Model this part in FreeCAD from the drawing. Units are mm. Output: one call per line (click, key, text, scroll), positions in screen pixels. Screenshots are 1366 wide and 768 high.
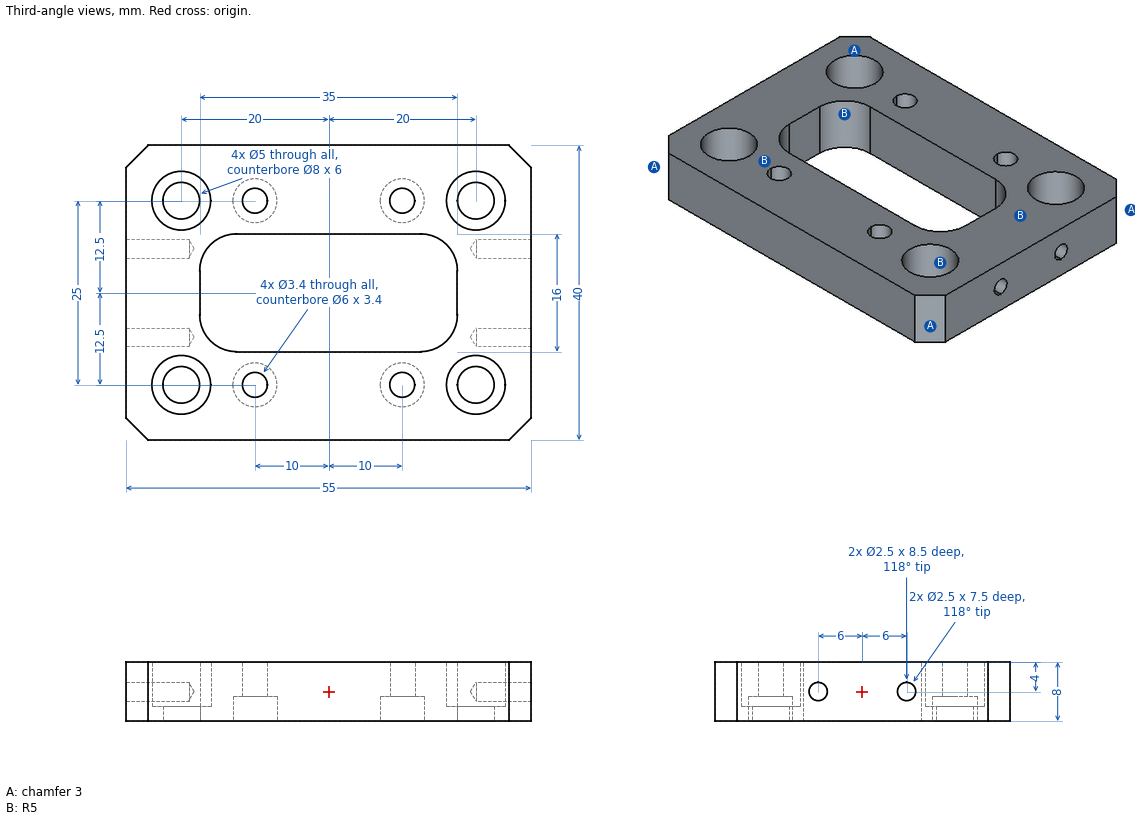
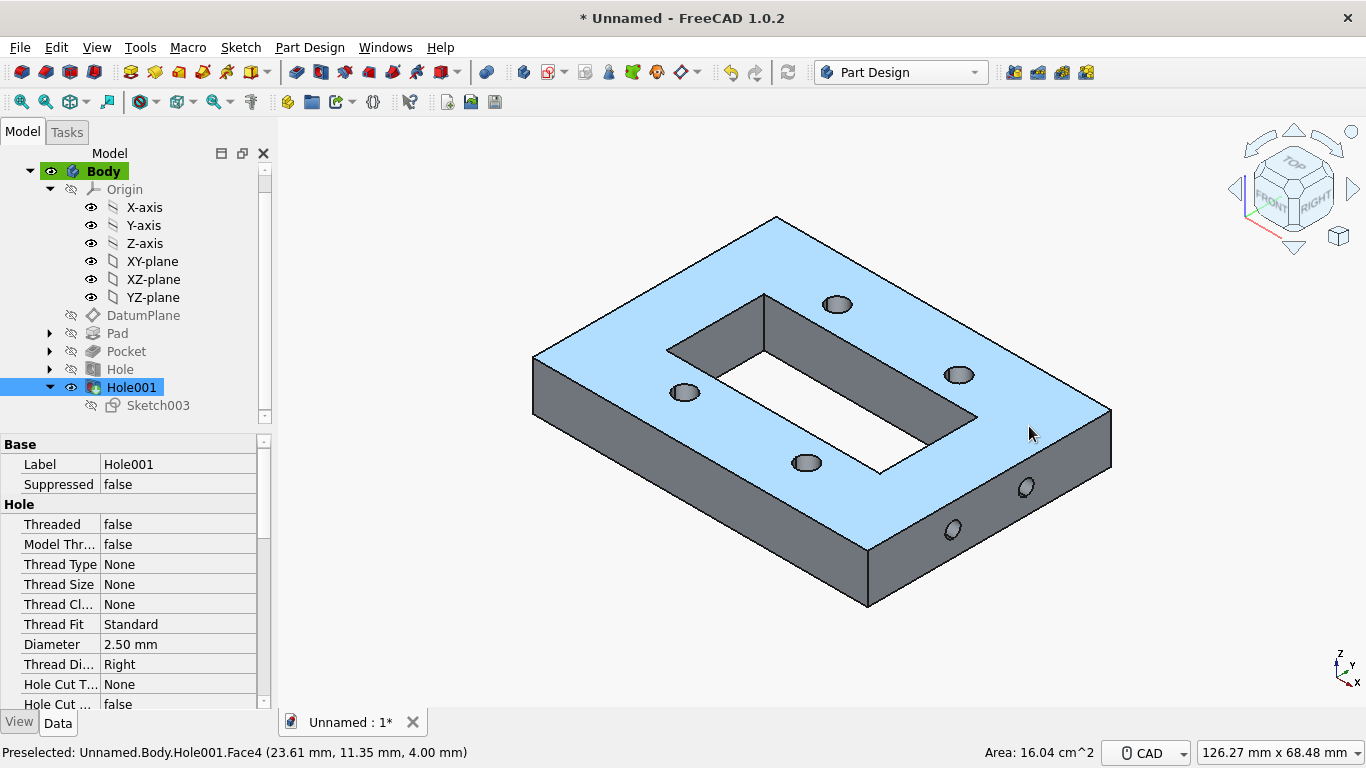
click(548, 72)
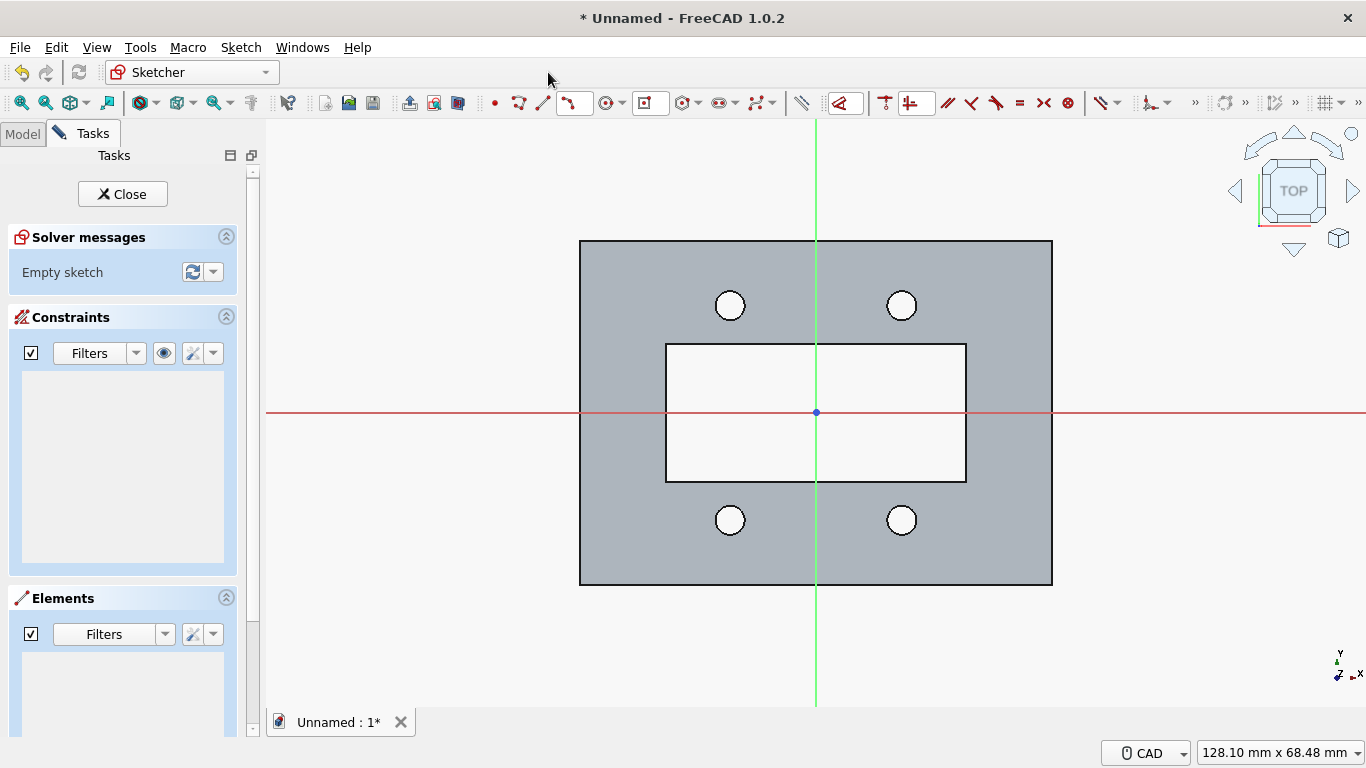
scroll(955, 413, up, 2)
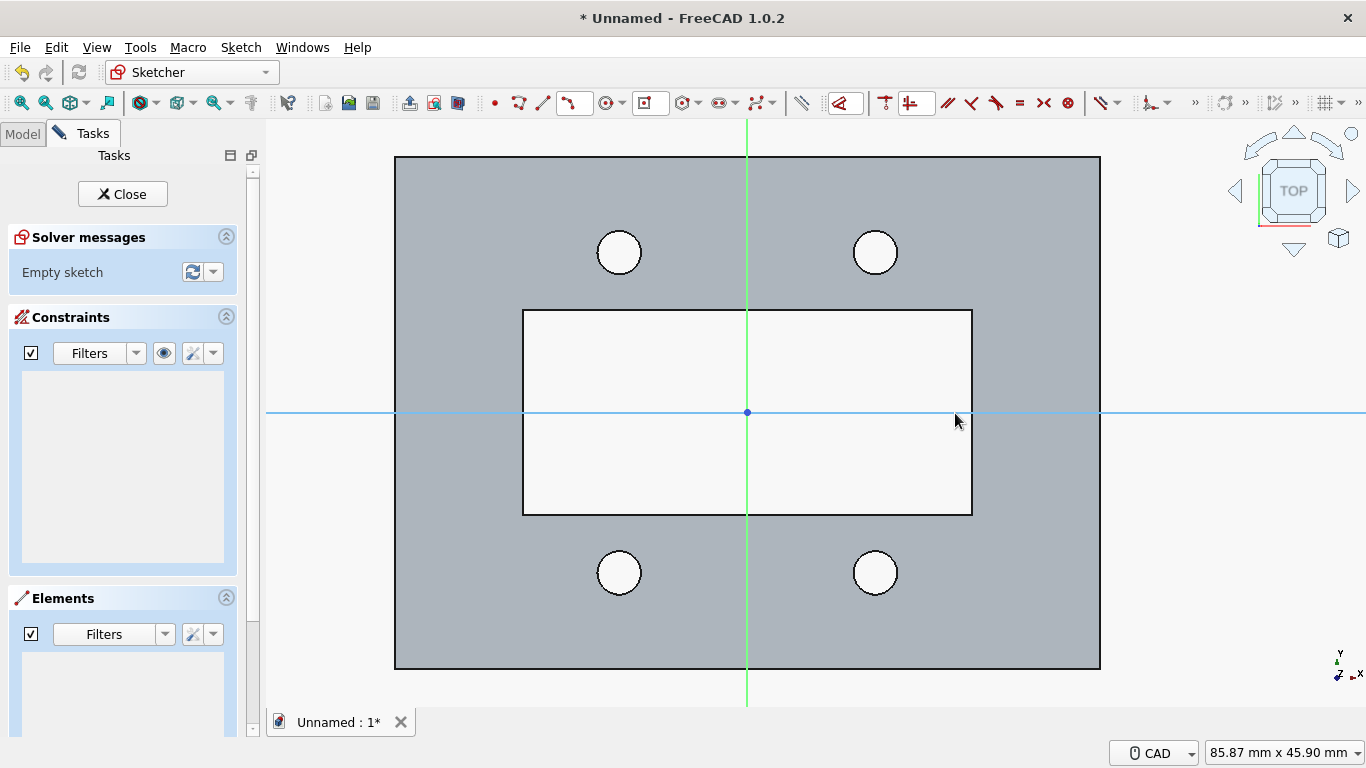
click(606, 104)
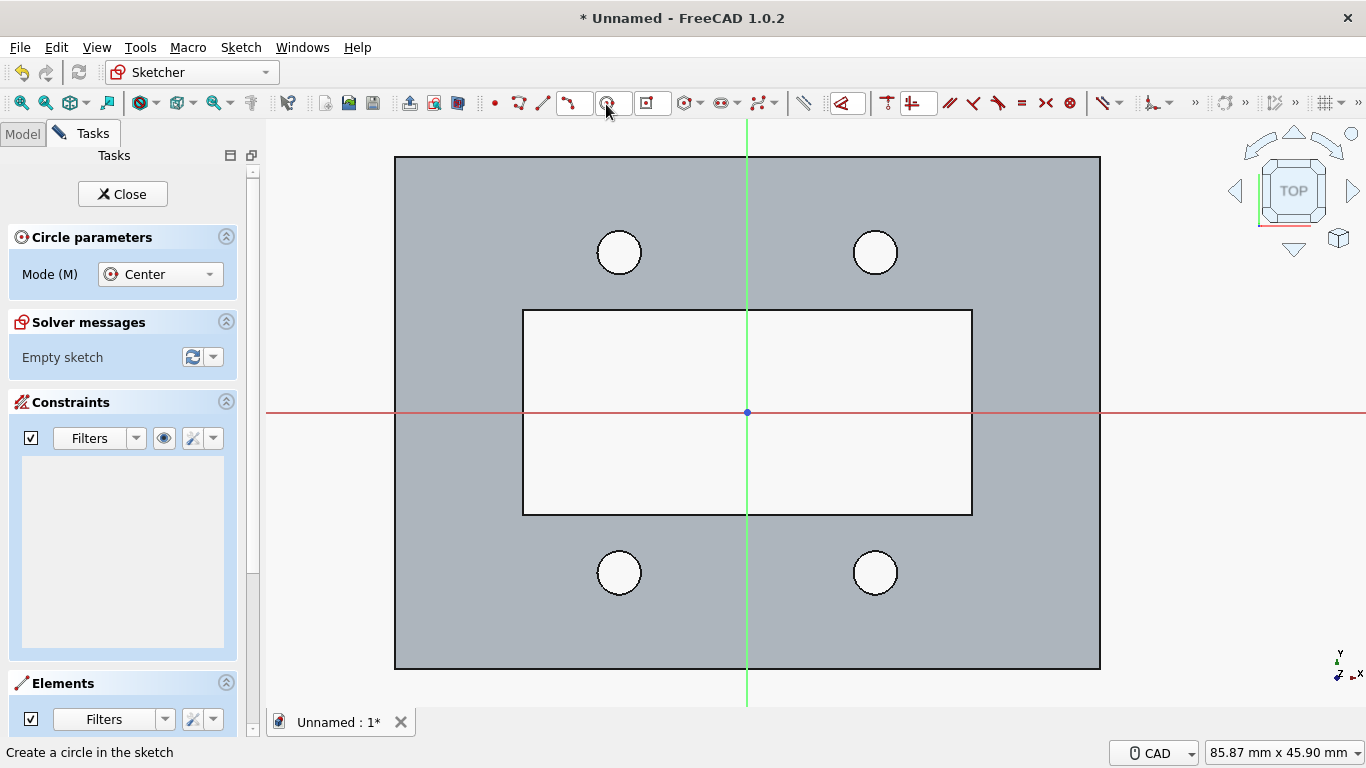
click(491, 253)
move(514, 230)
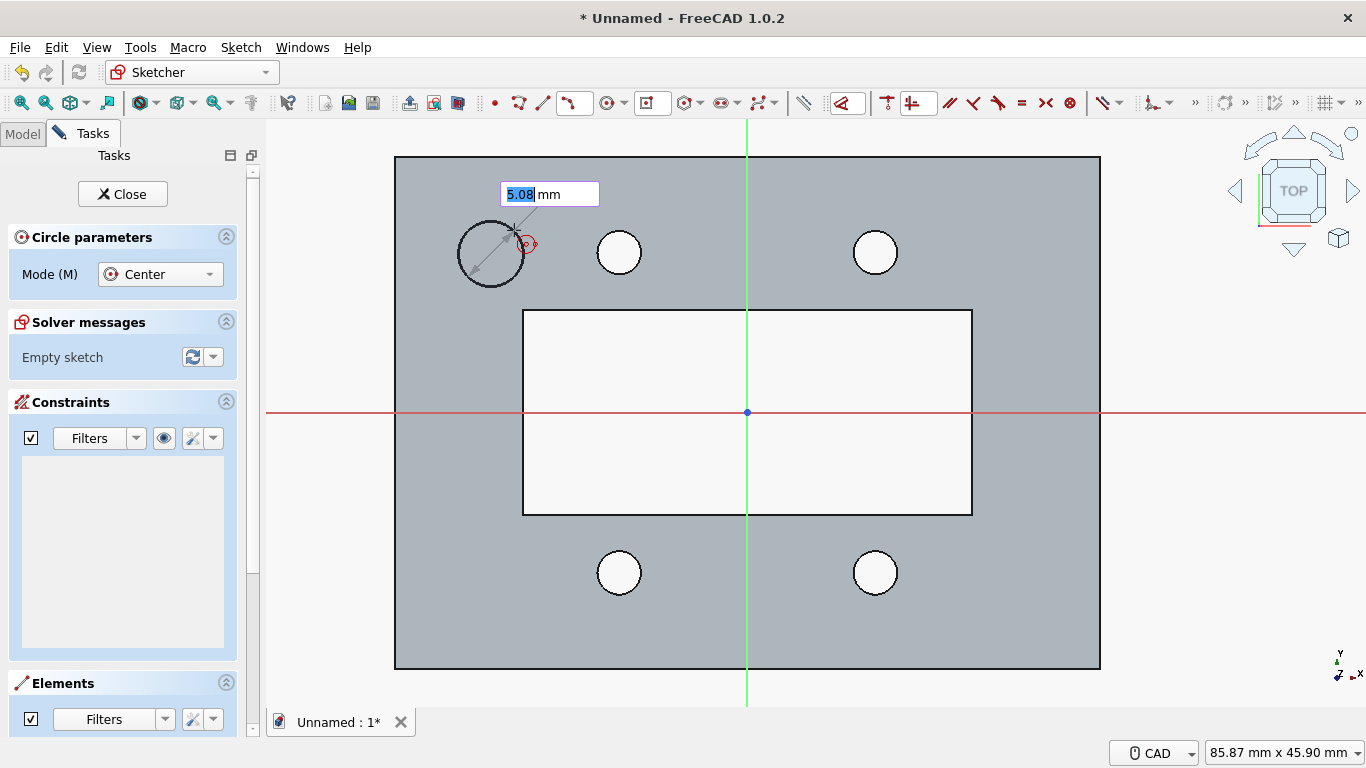
text(5)
key(Return)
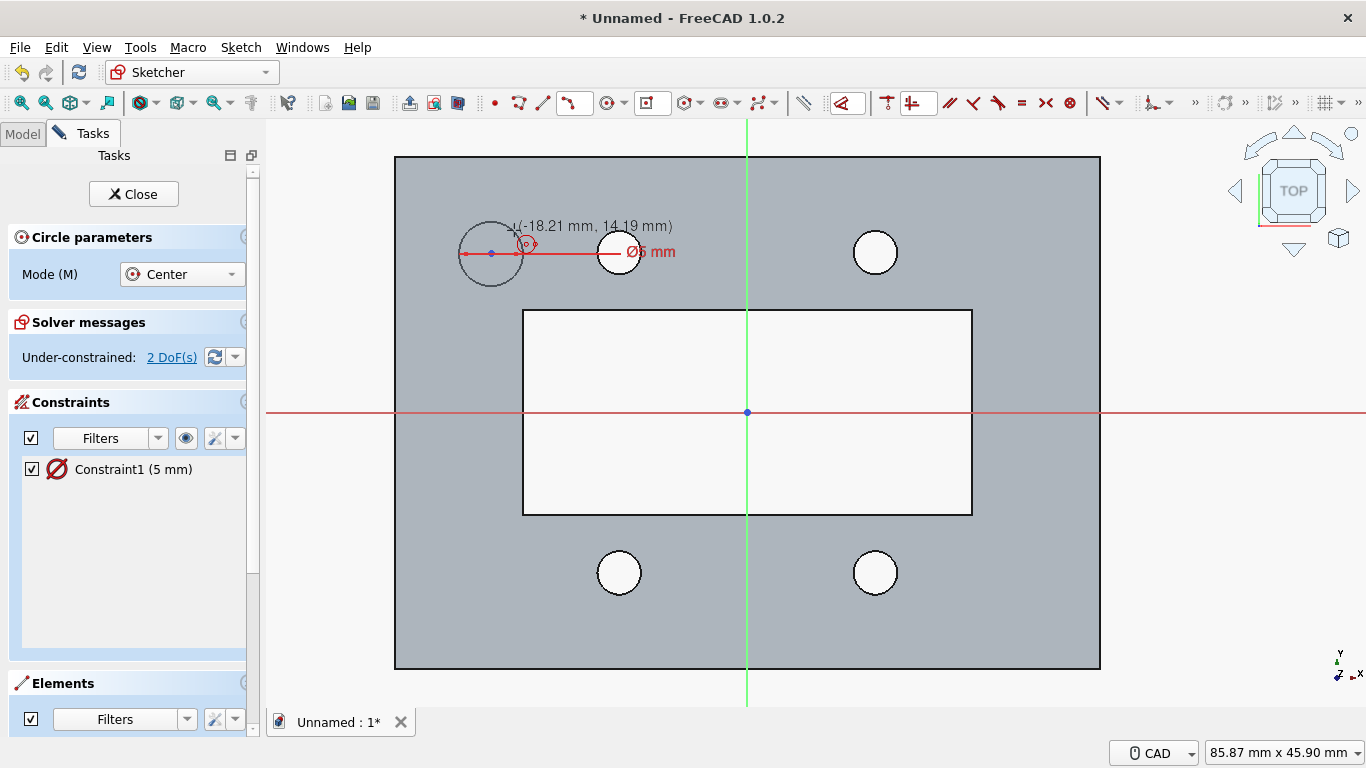
click(491, 573)
move(514, 550)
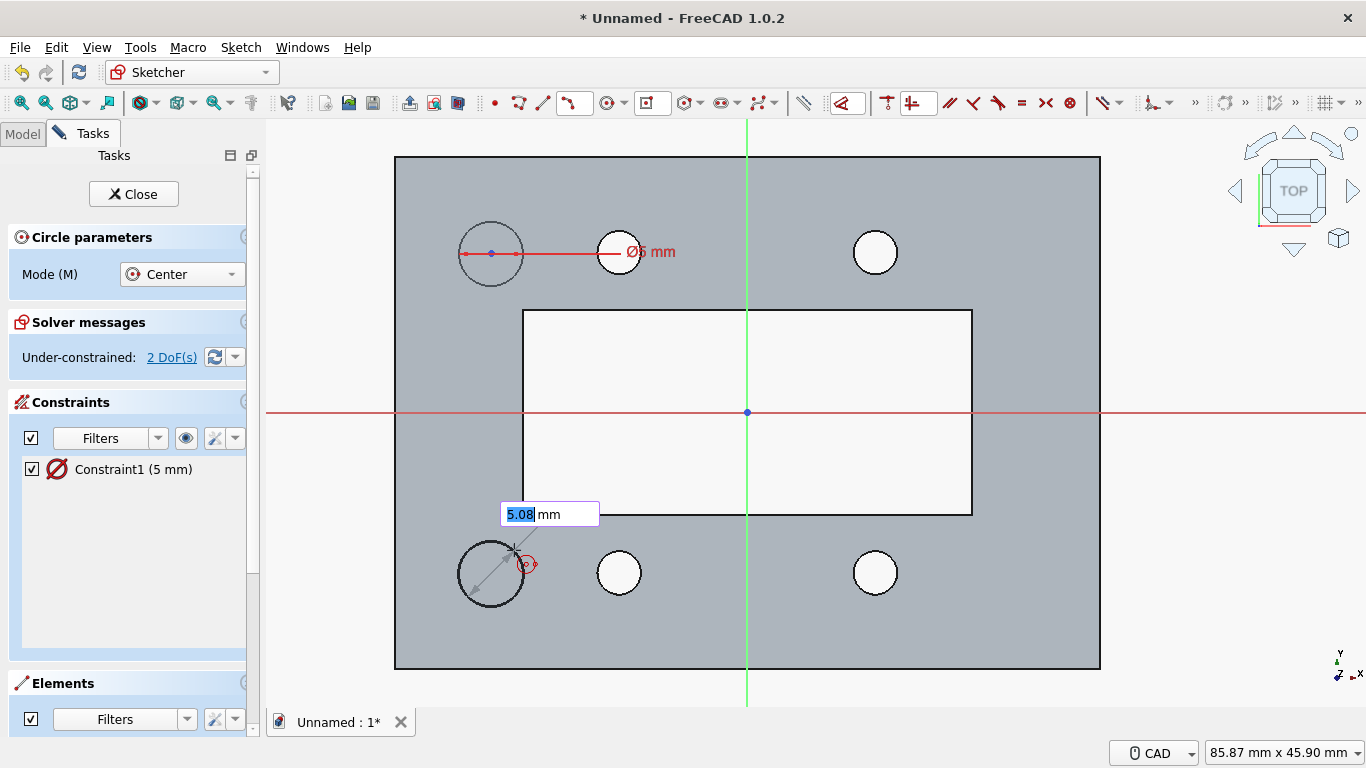
text(5)
key(Return)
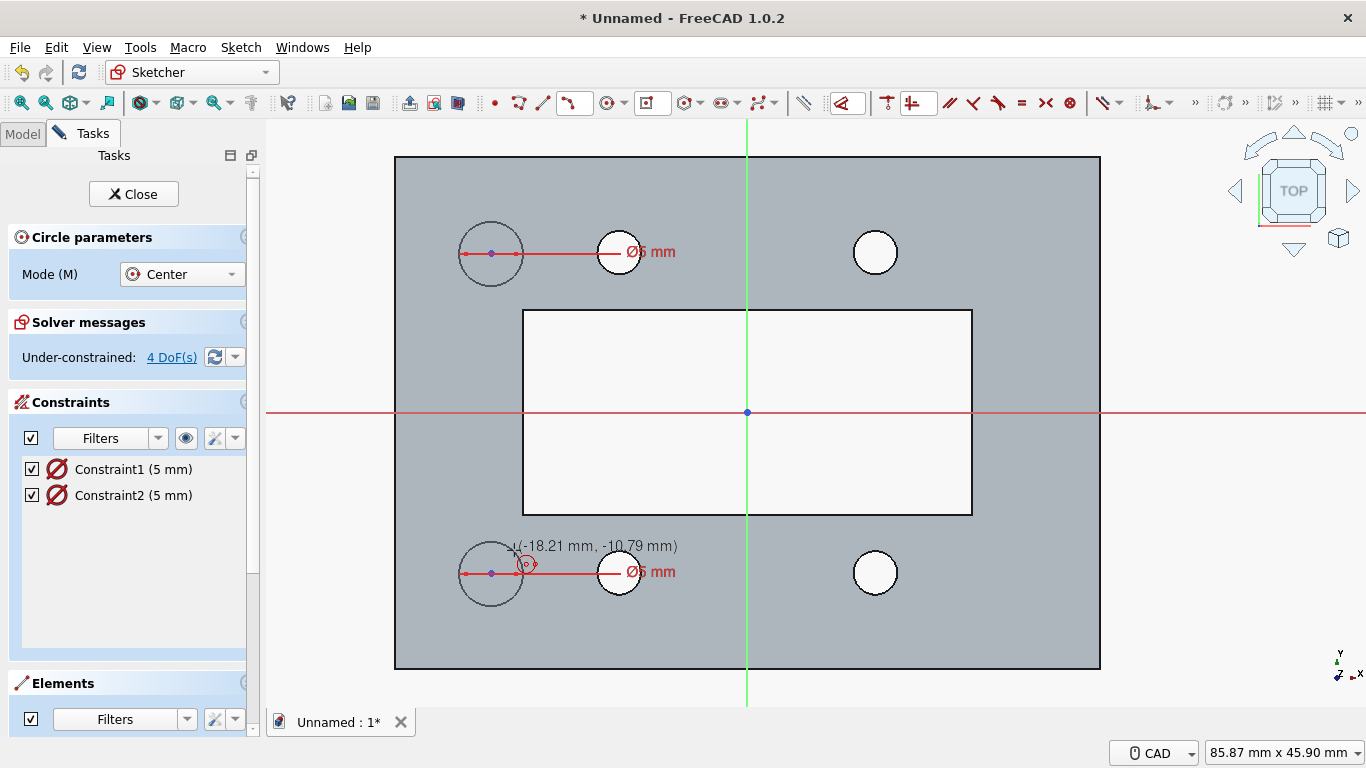
click(1004, 253)
move(1026, 230)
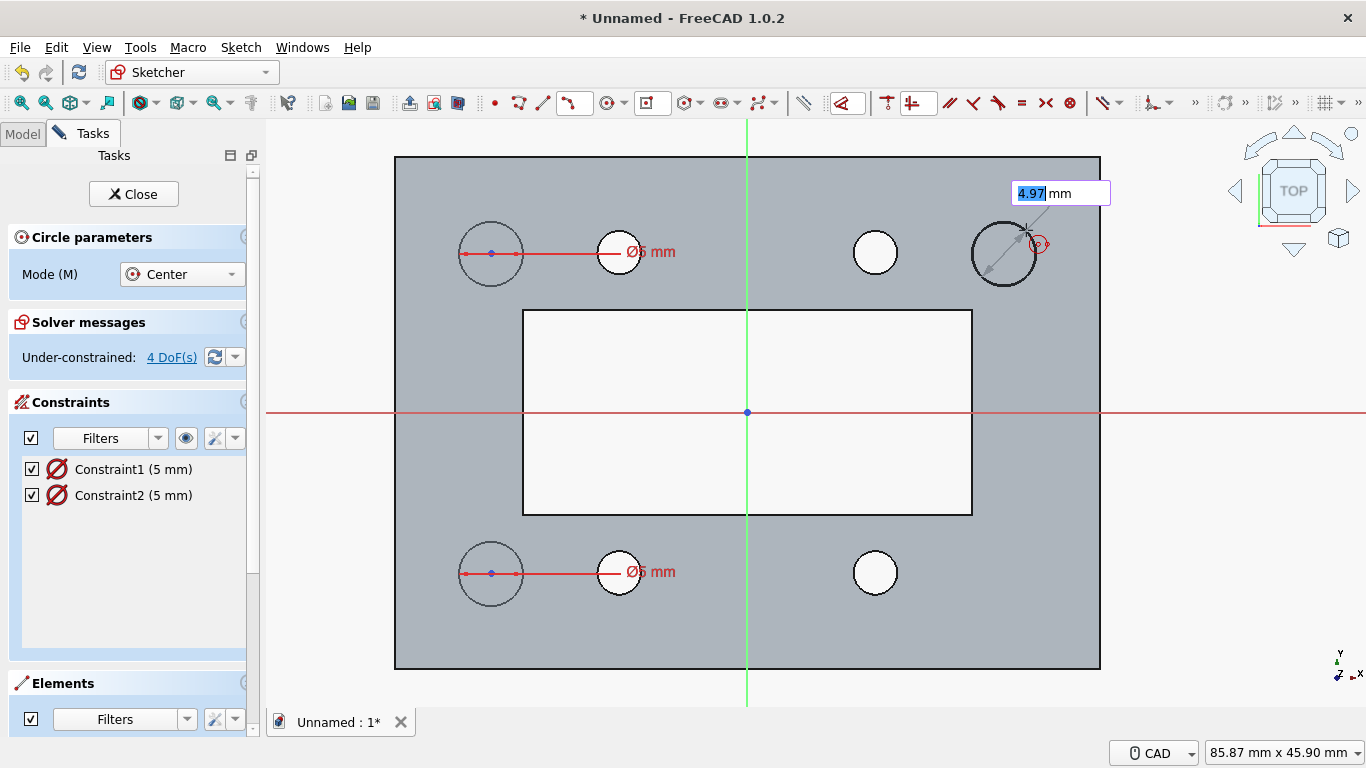
text(5)
key(Return)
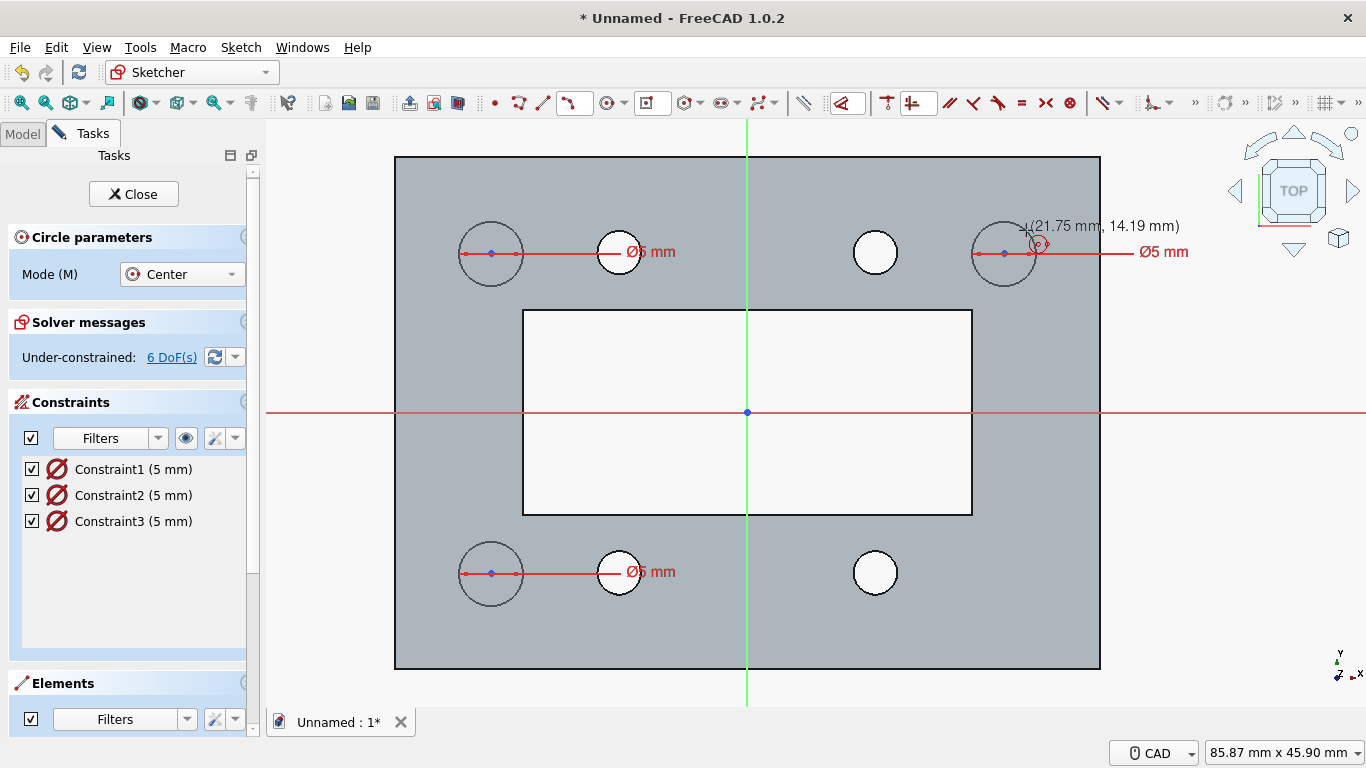
click(1004, 573)
move(1026, 550)